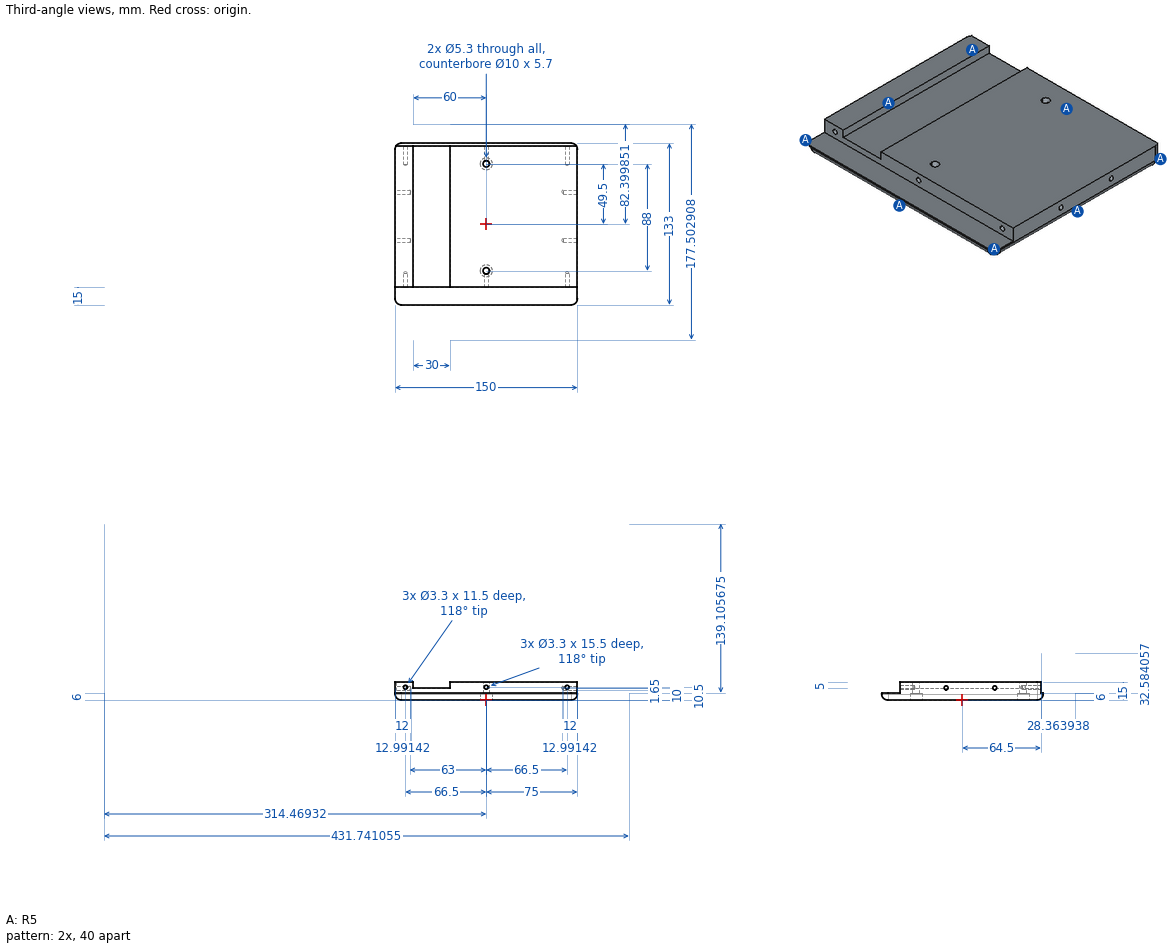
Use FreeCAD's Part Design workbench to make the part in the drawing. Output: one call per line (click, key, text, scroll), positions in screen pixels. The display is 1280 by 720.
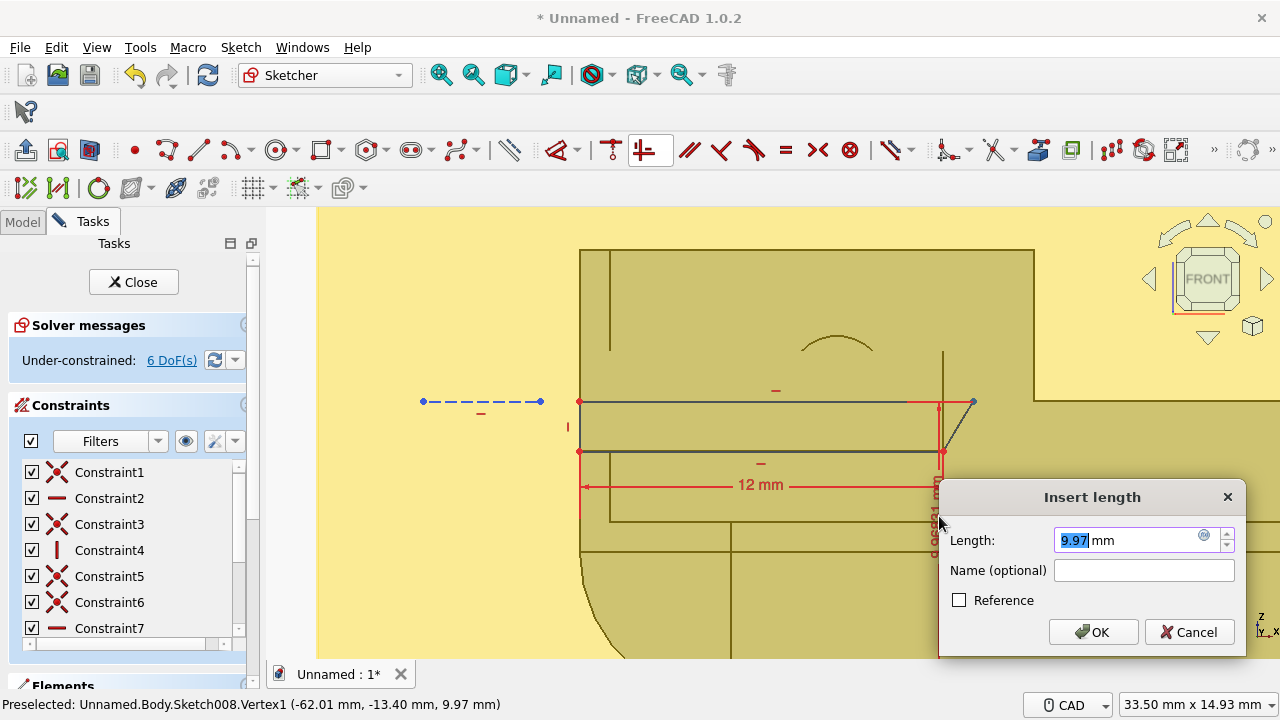
text(10)
key(Return)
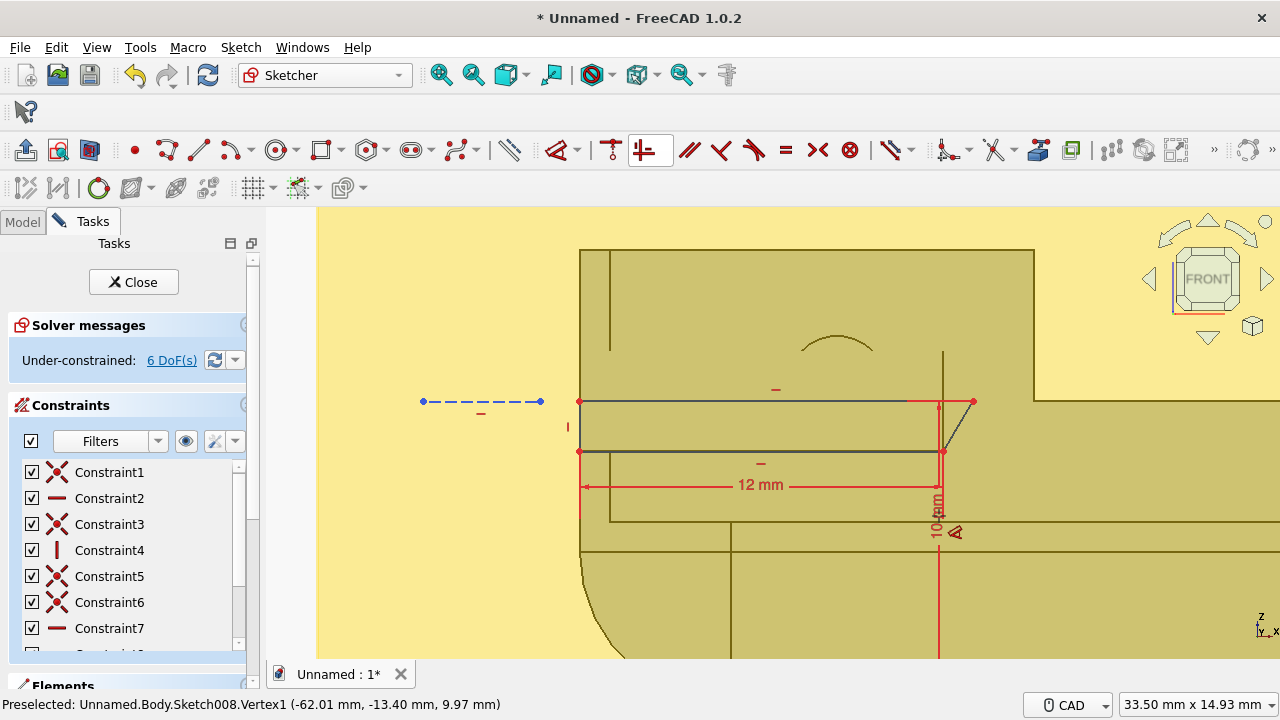
click(943, 452)
click(1029, 418)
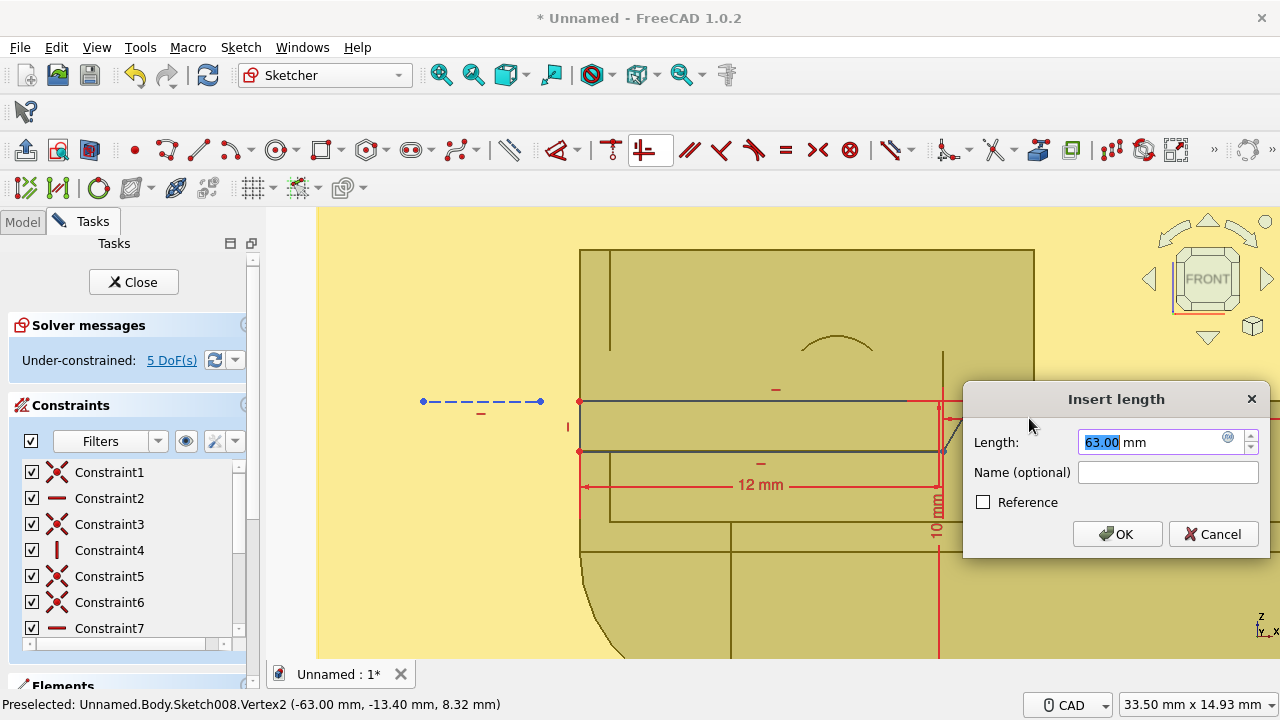
text(63)
key(Return)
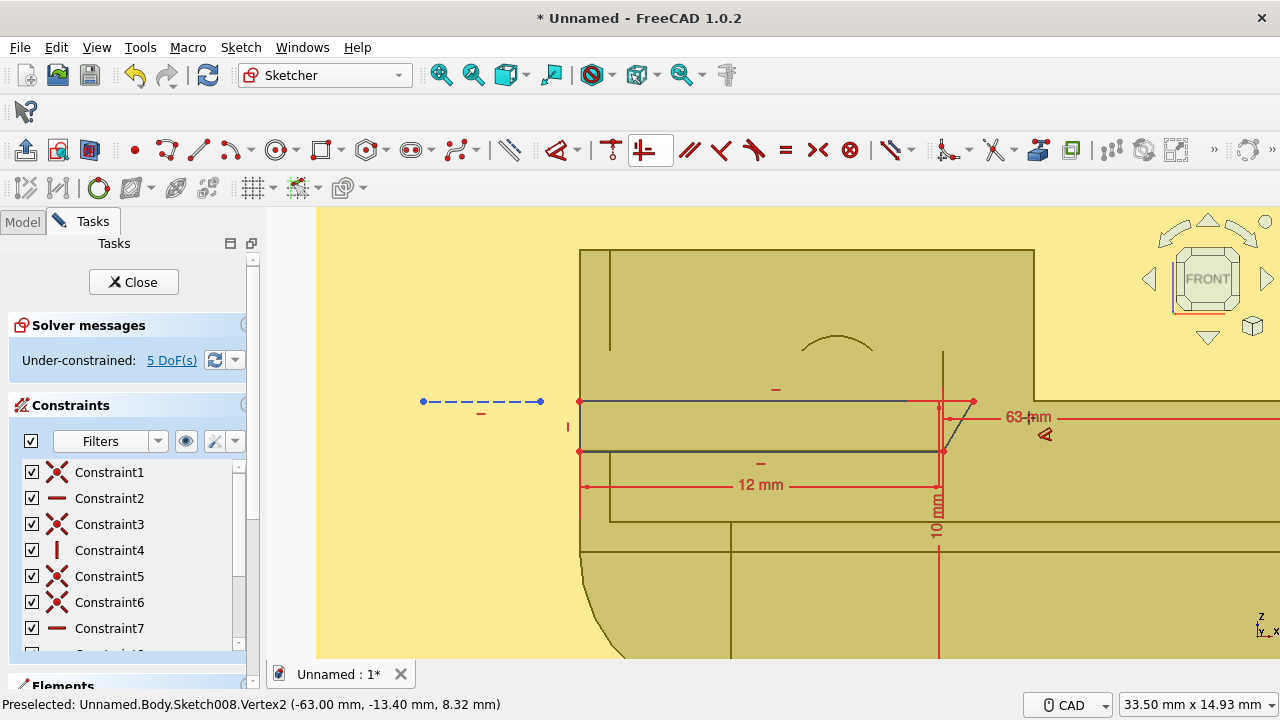
click(541, 402)
click(507, 516)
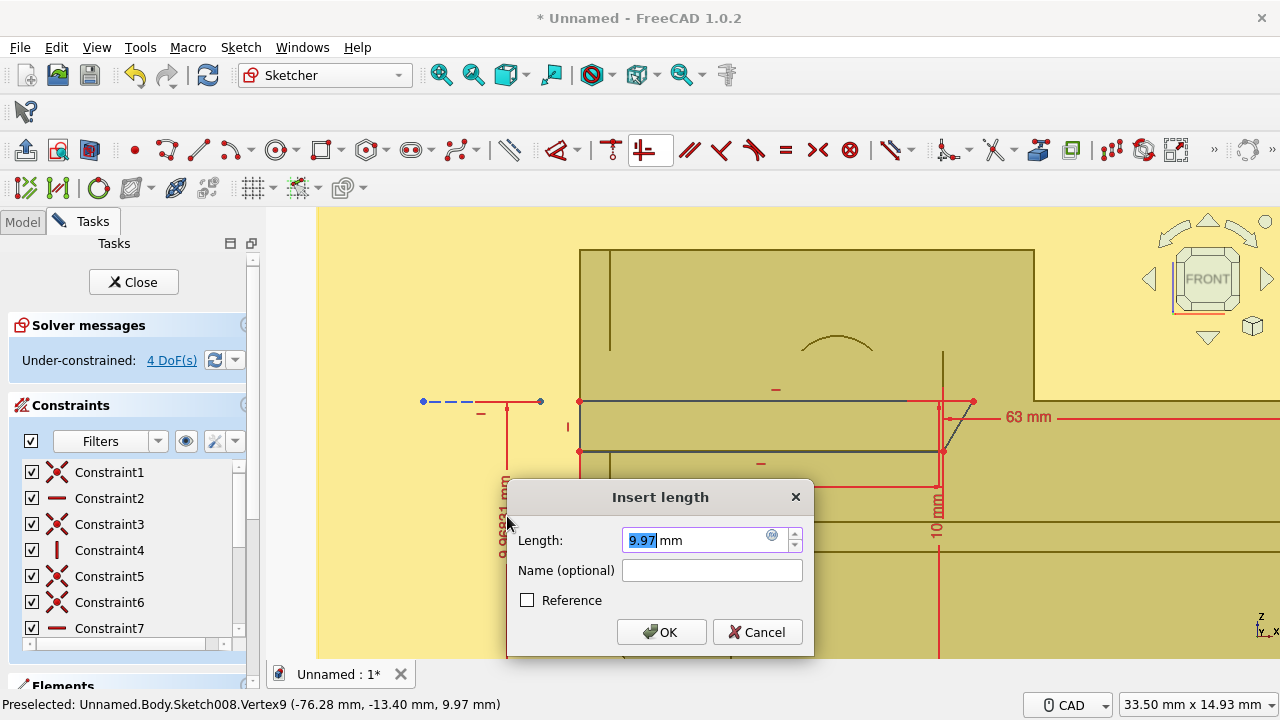
text(10)
key(Return)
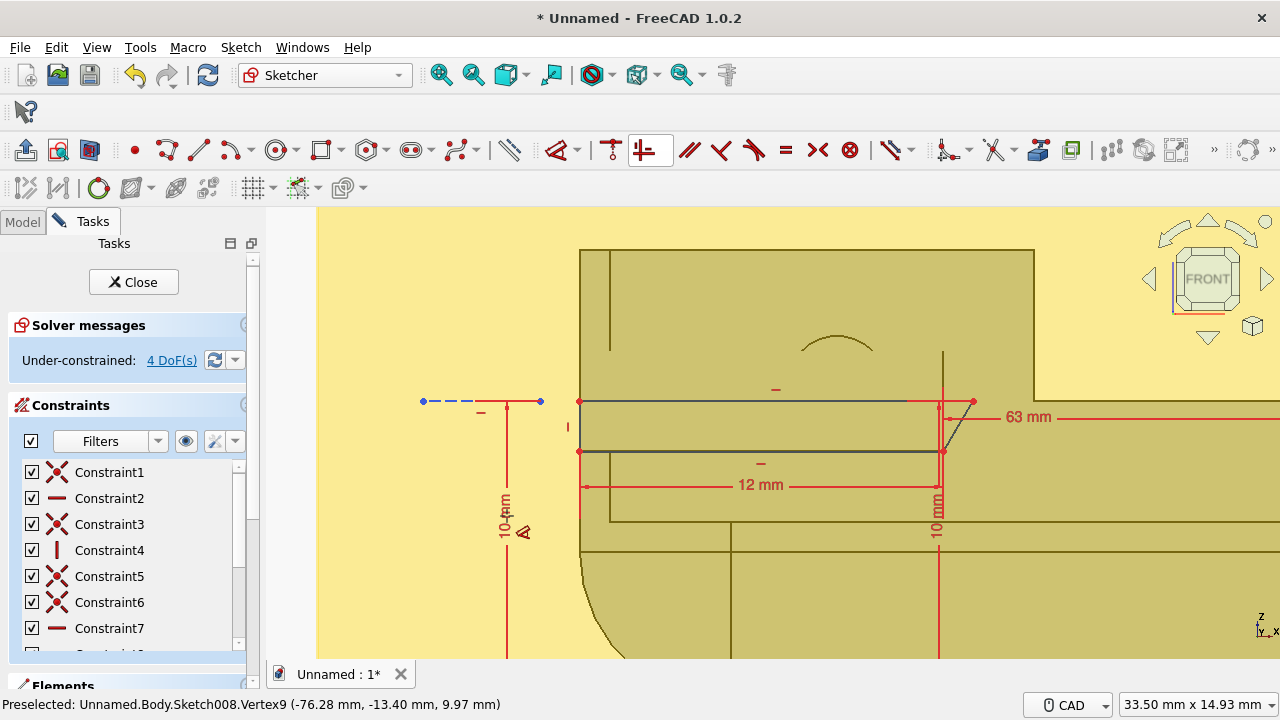
click(580, 437)
click(546, 427)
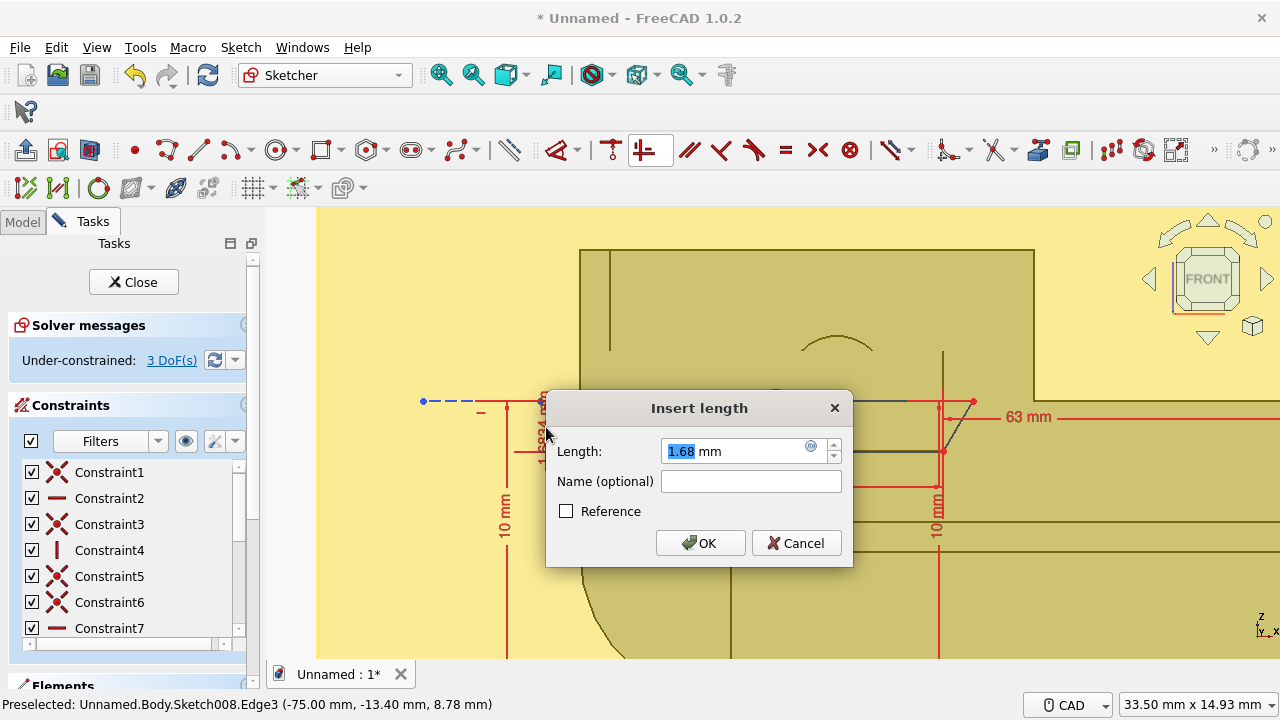
text(1.65)
key(Return)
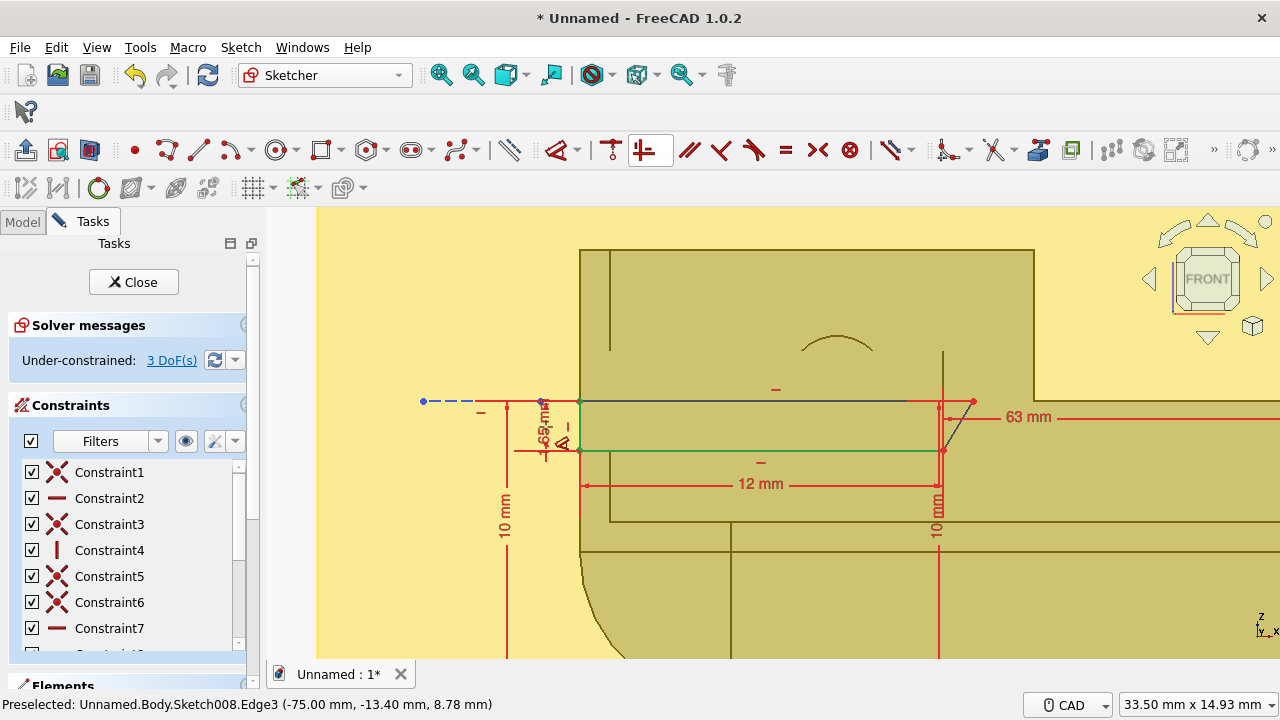
click(698, 401)
click(776, 367)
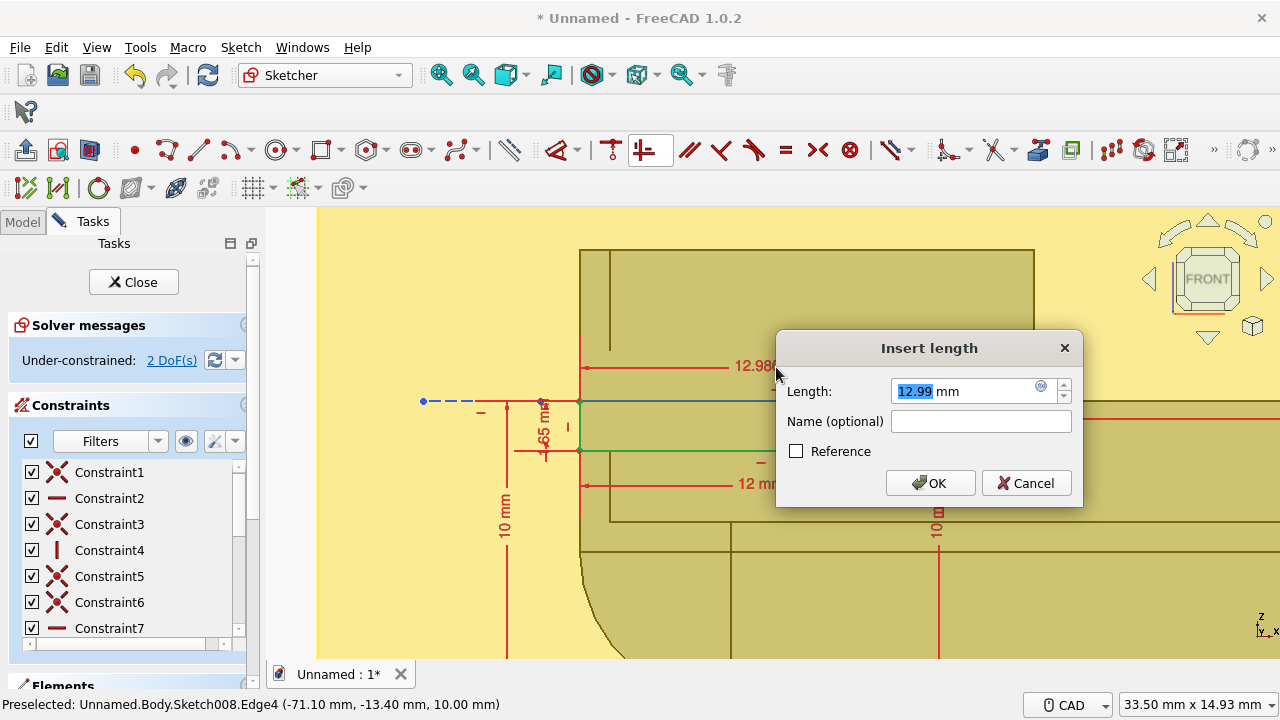
text(12.99142)
key(Return)
key(Escape)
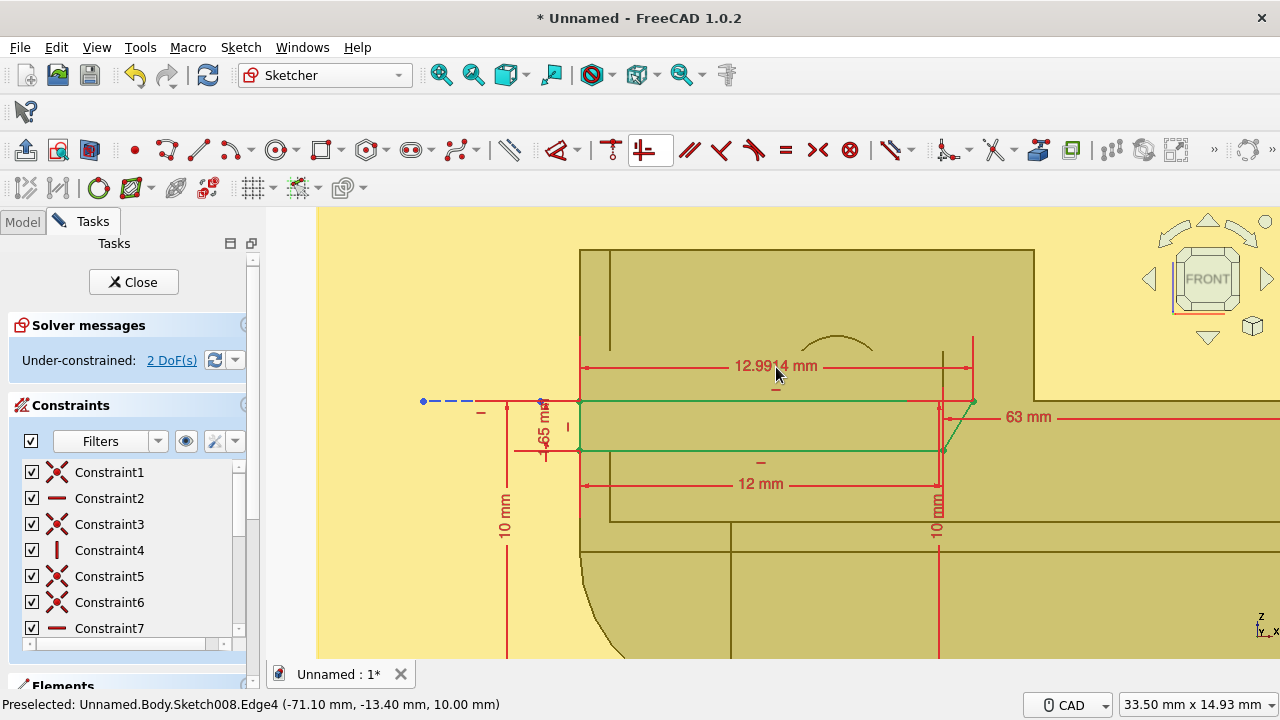
click(134, 282)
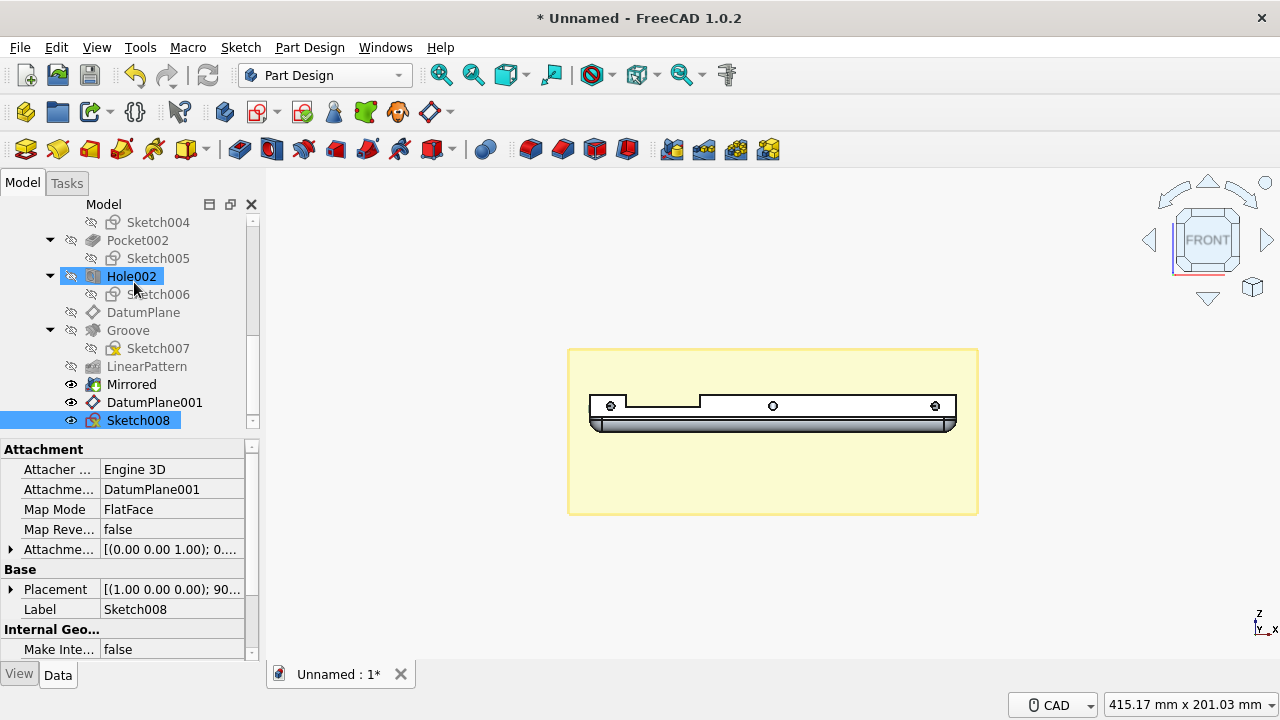
click(304, 150)